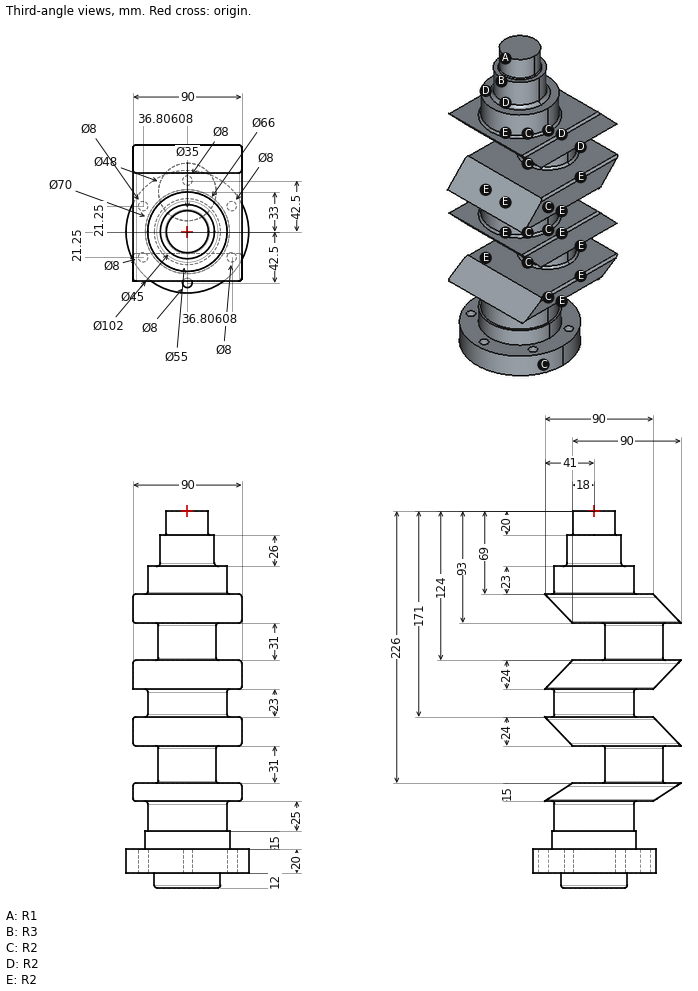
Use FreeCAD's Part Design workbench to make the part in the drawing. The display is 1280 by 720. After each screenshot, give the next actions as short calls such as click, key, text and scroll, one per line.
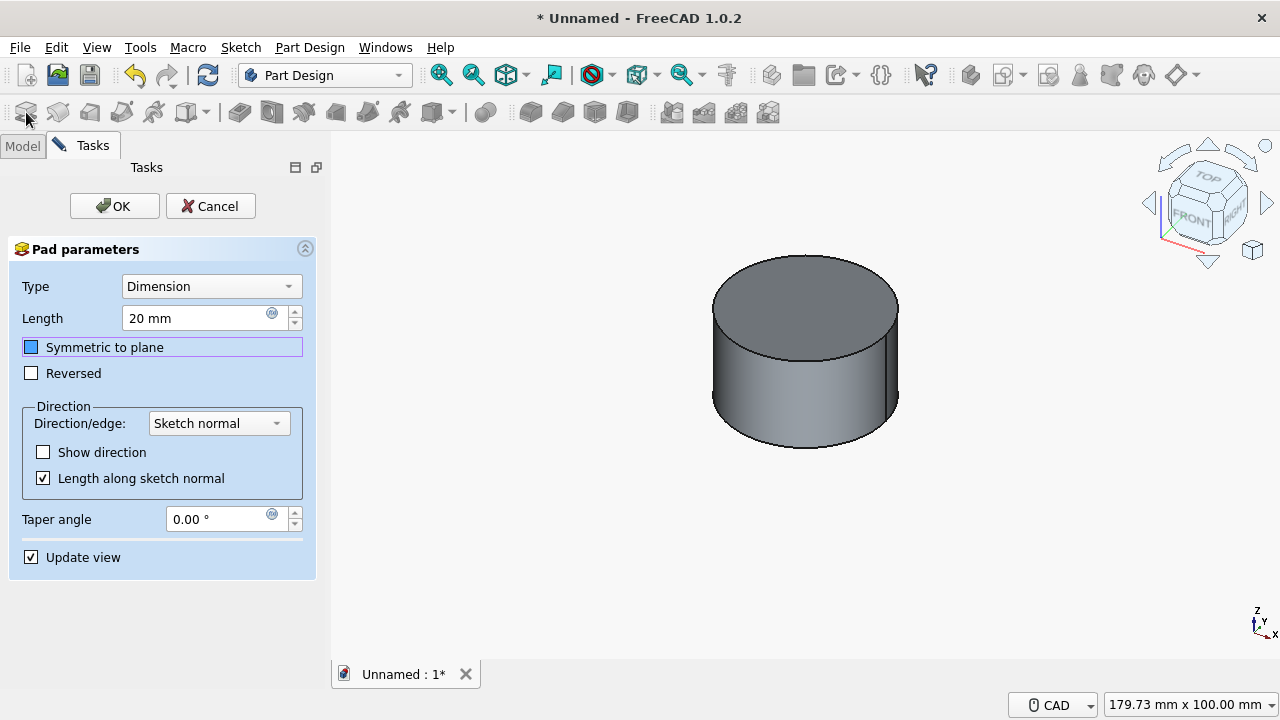
click(30, 373)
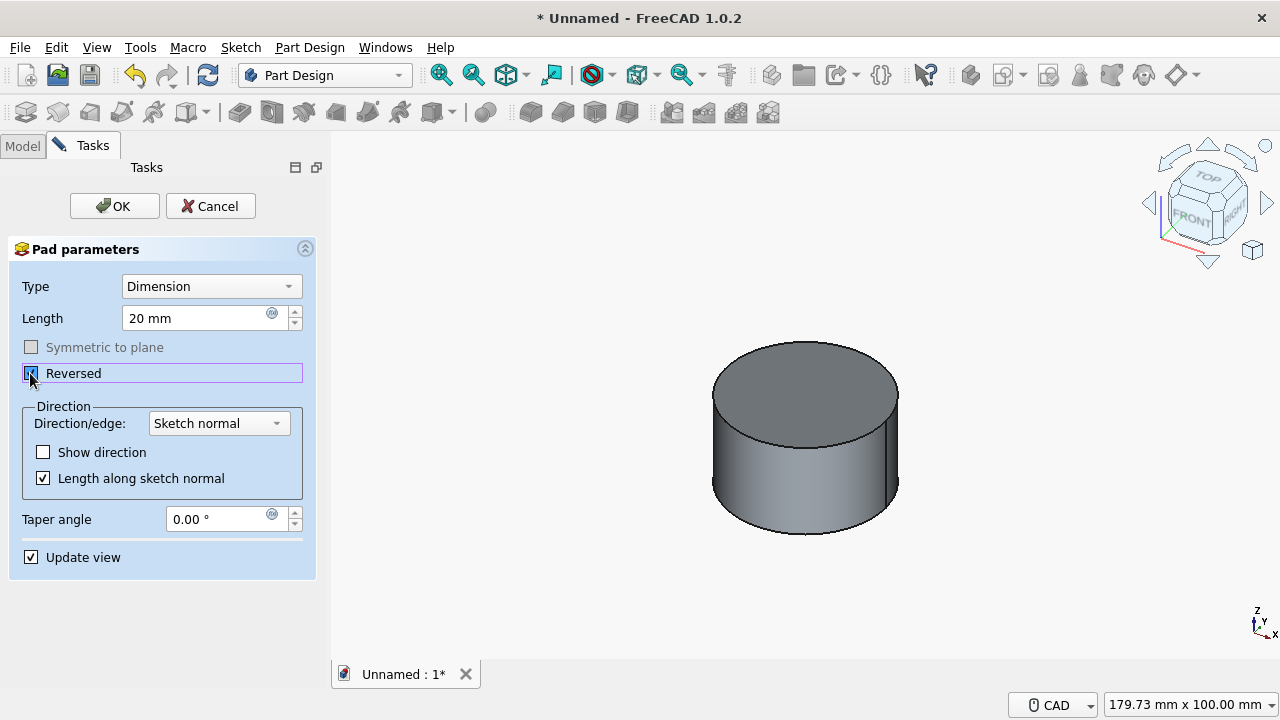
click(115, 206)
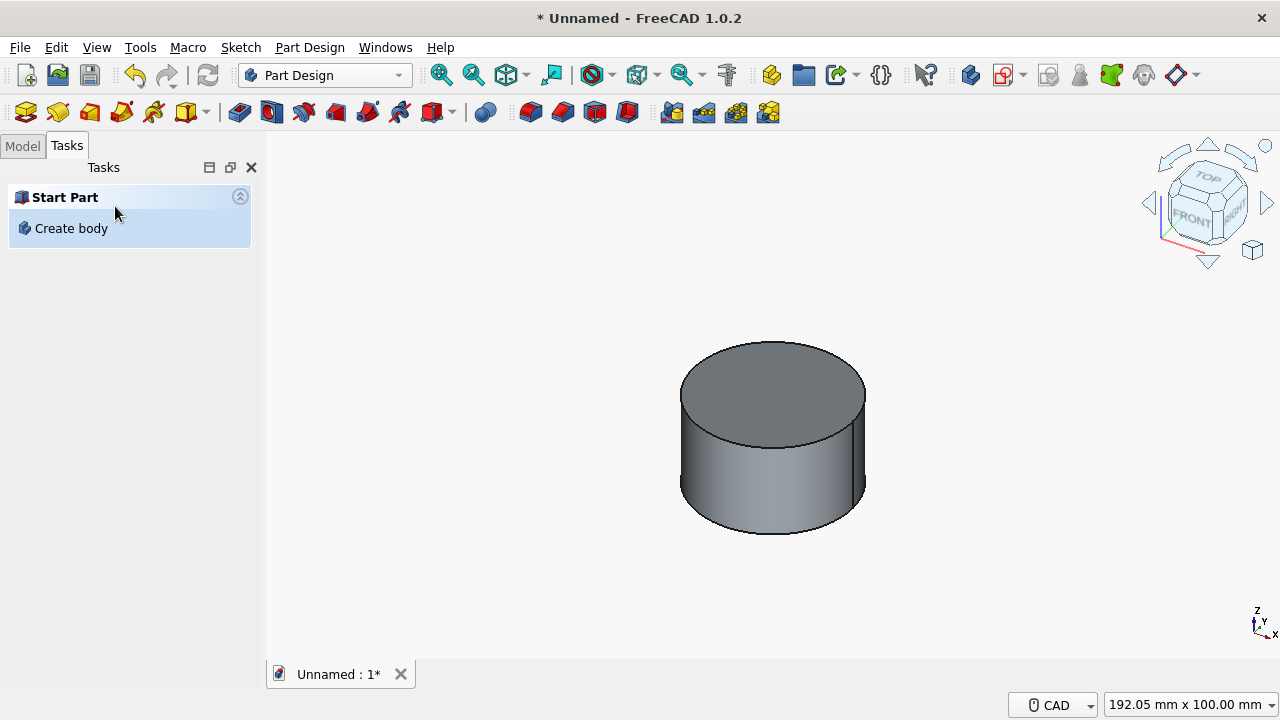
click(442, 76)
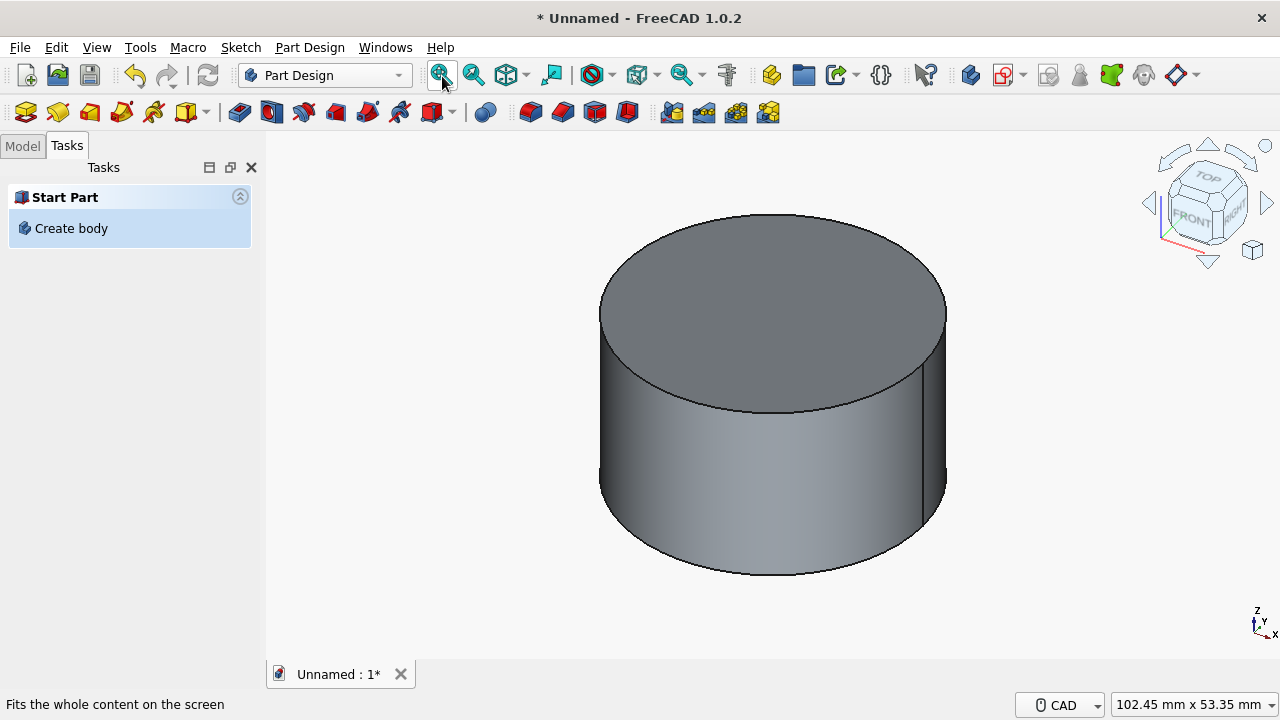
key(5)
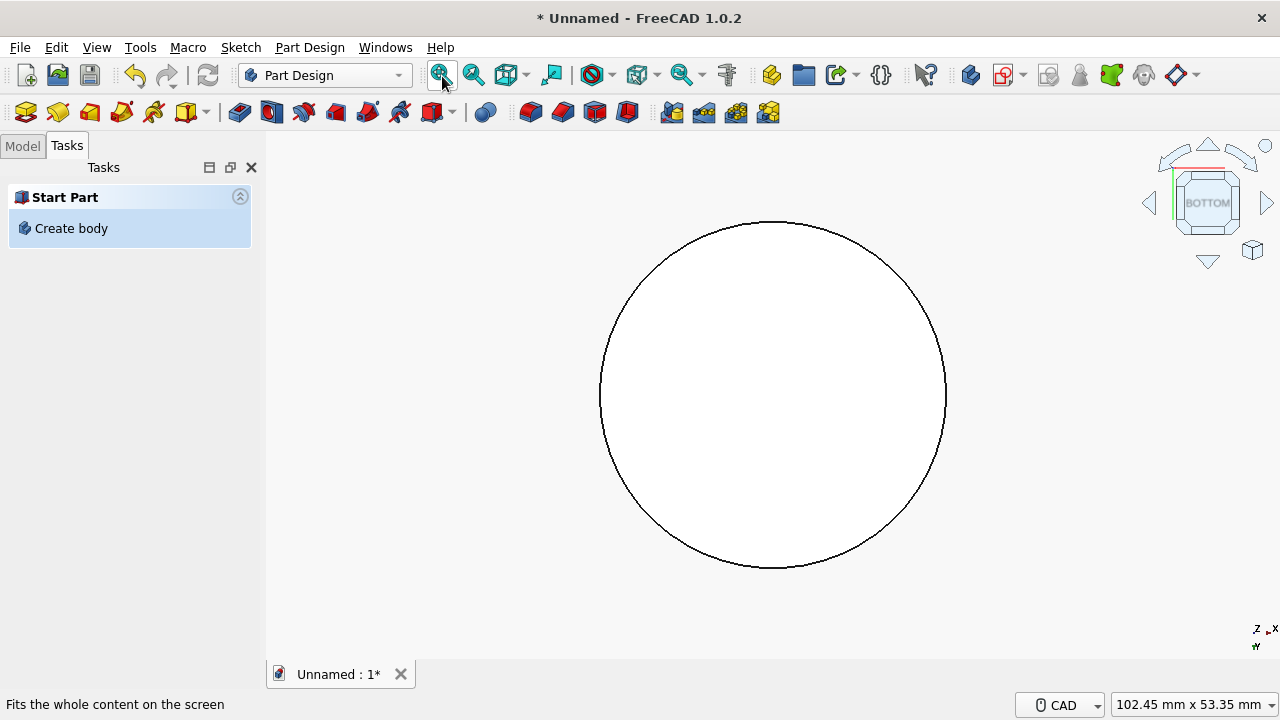
click(773, 394)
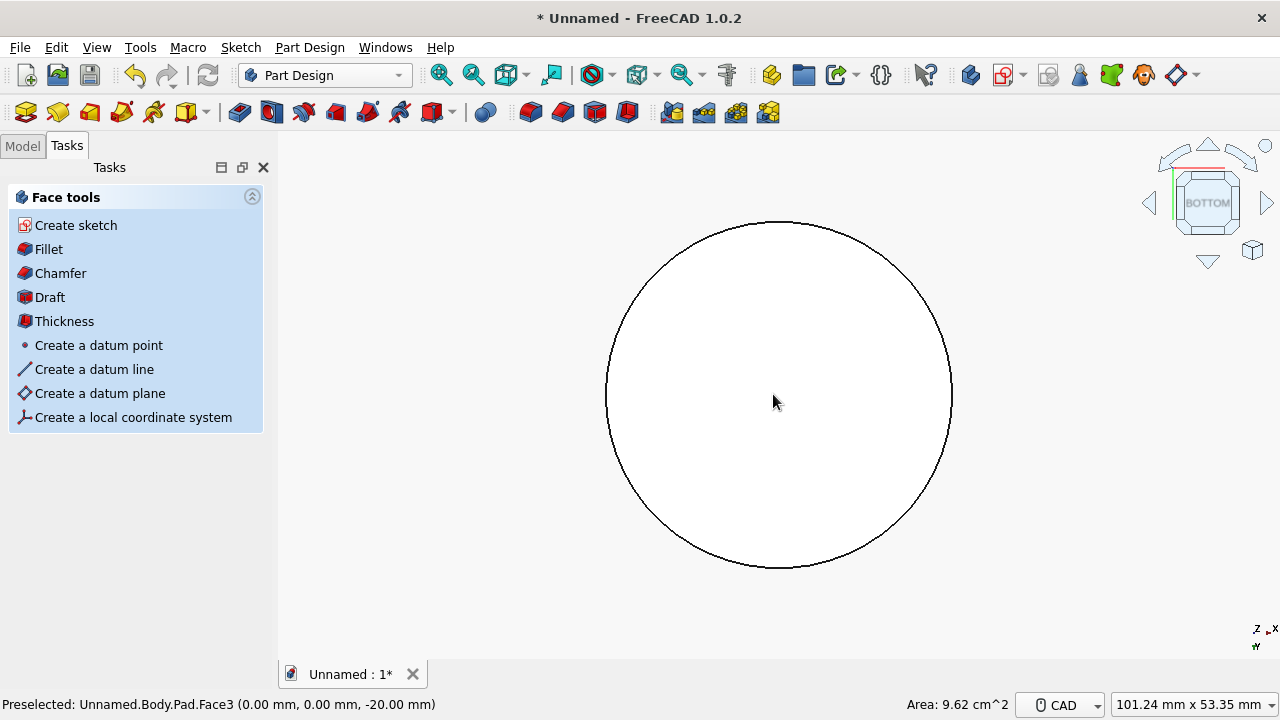
click(1004, 76)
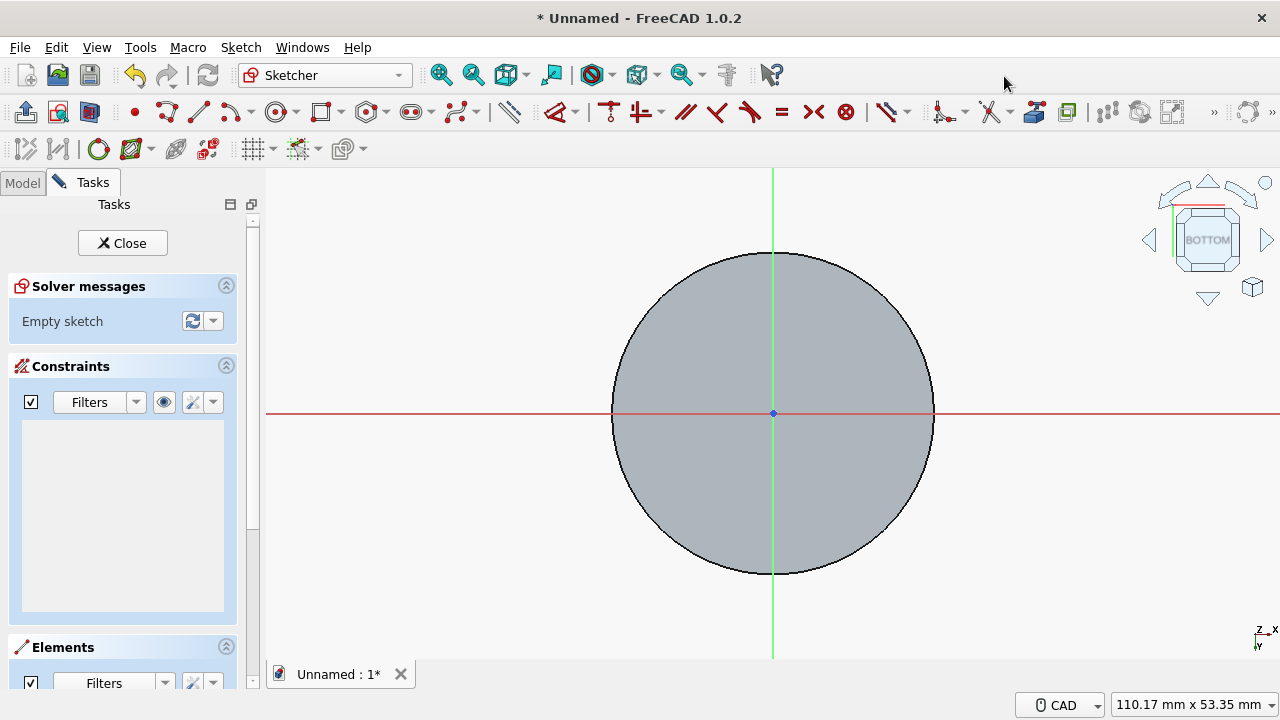
scroll(395, 413, down, 1)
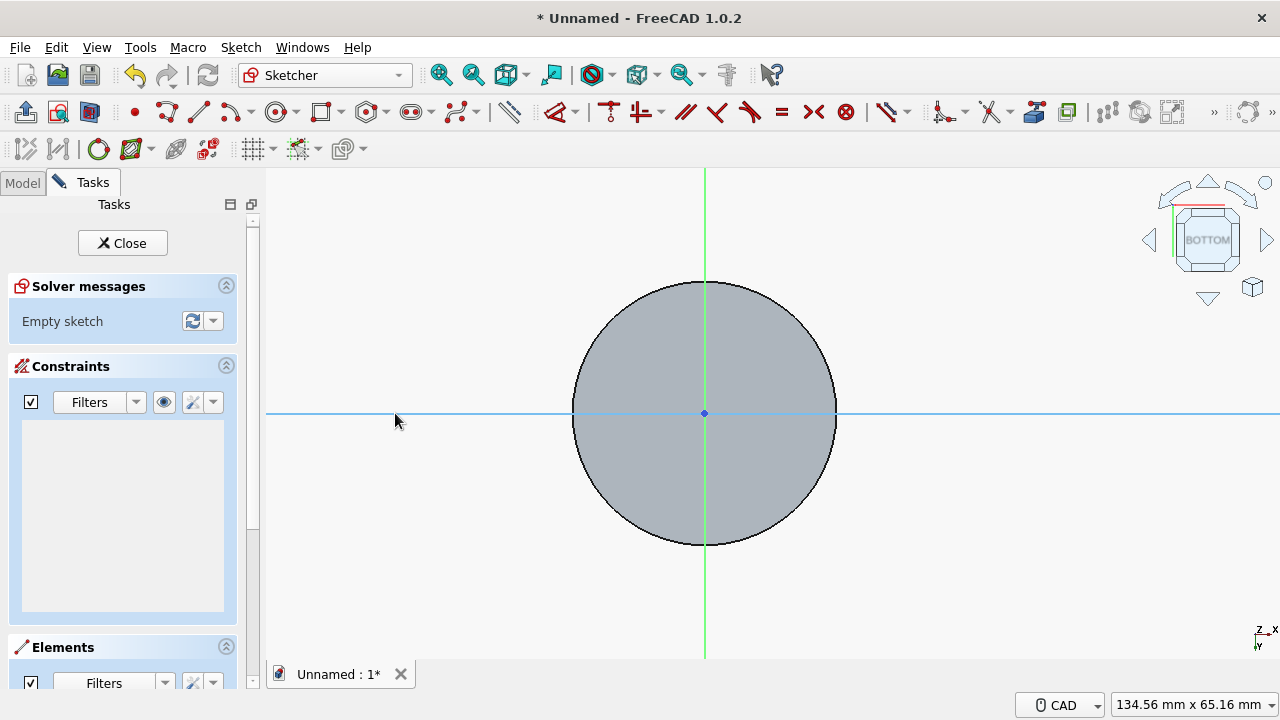
click(276, 112)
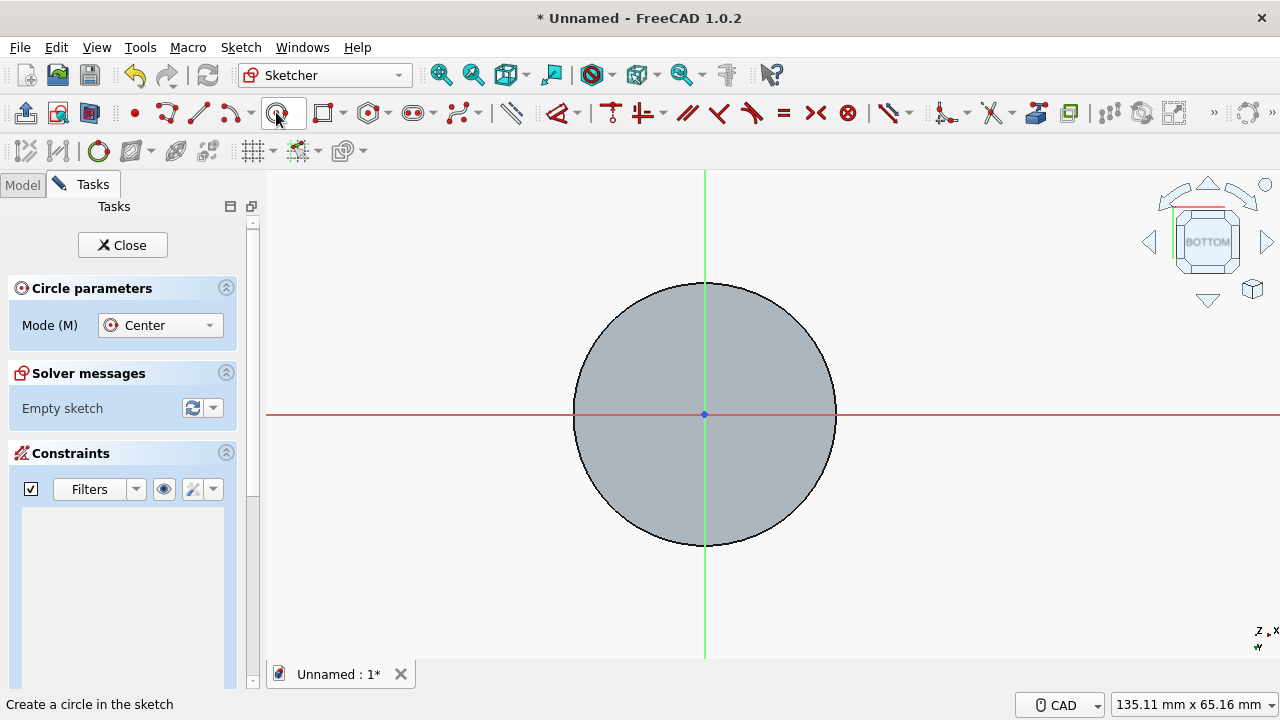
click(705, 414)
move(824, 295)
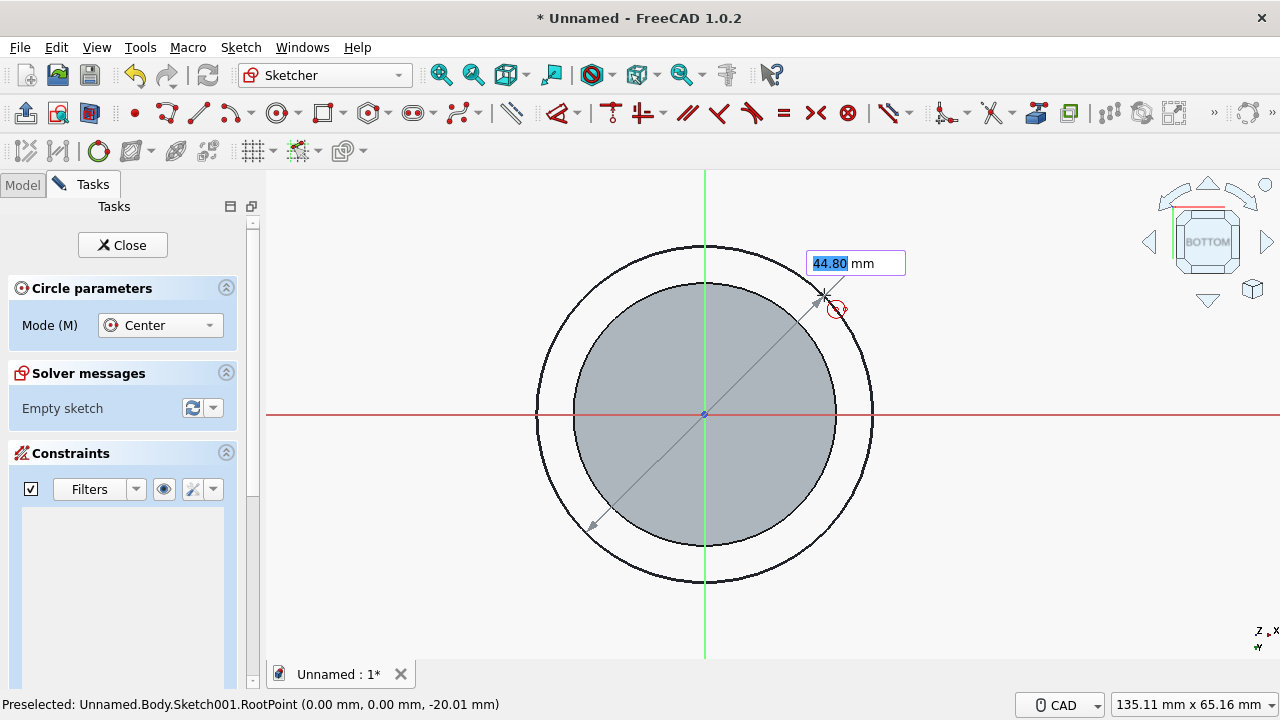
text(45)
key(Return)
key(Escape)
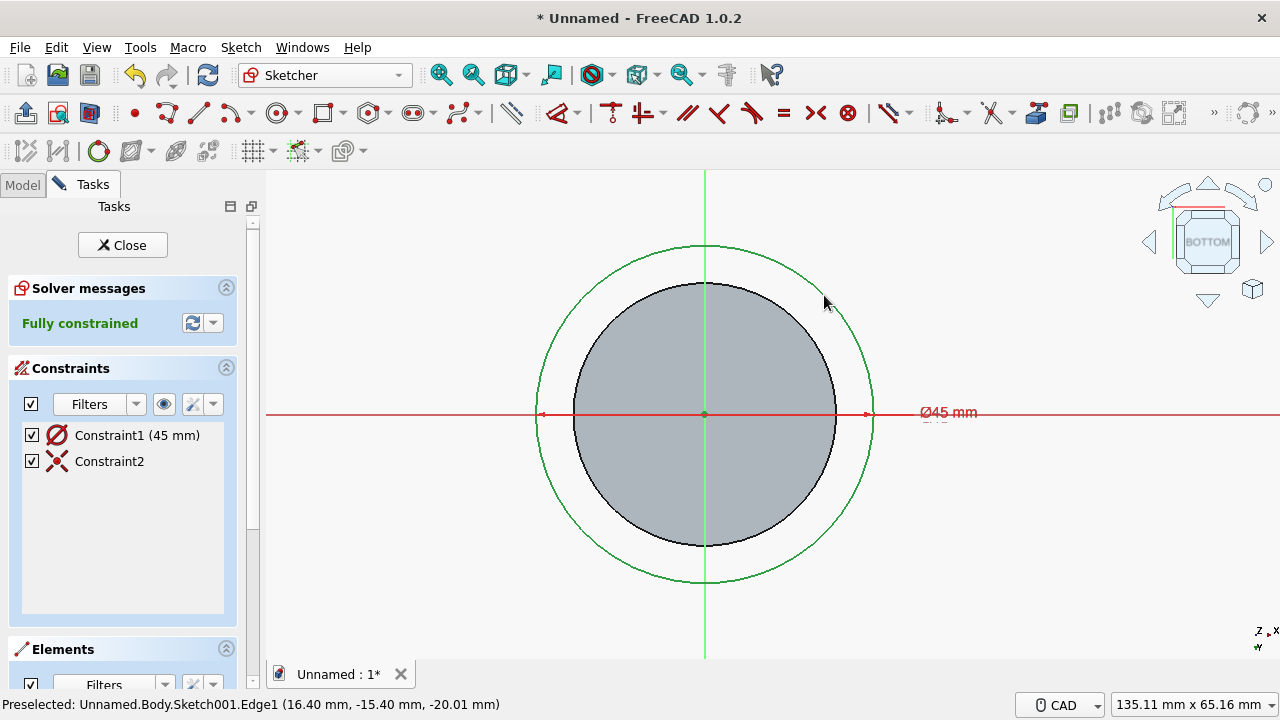
click(123, 245)